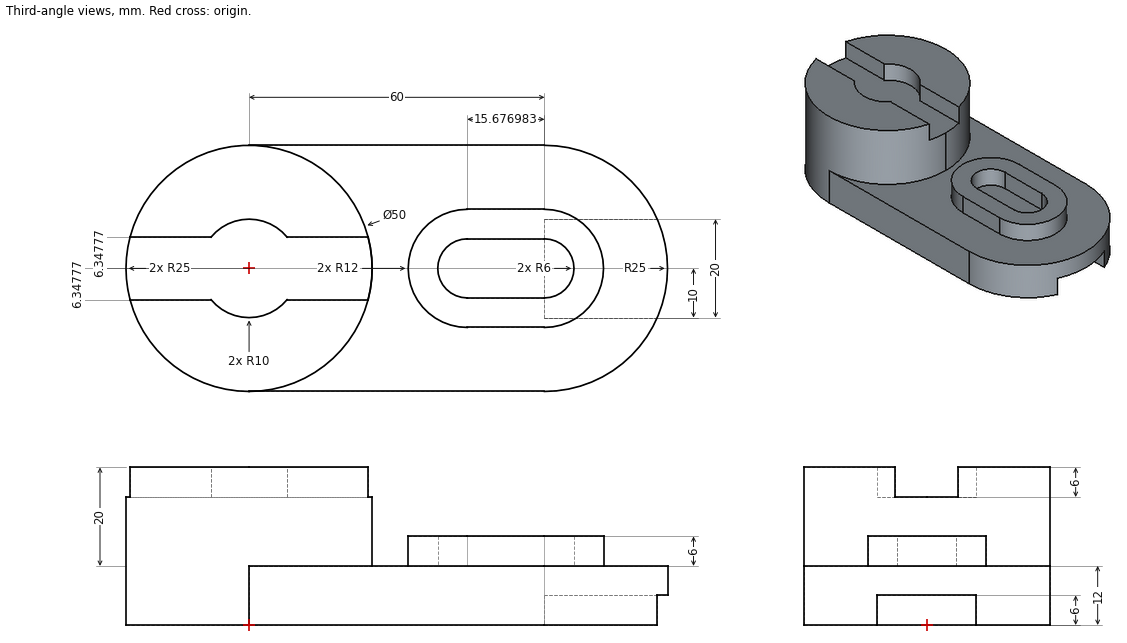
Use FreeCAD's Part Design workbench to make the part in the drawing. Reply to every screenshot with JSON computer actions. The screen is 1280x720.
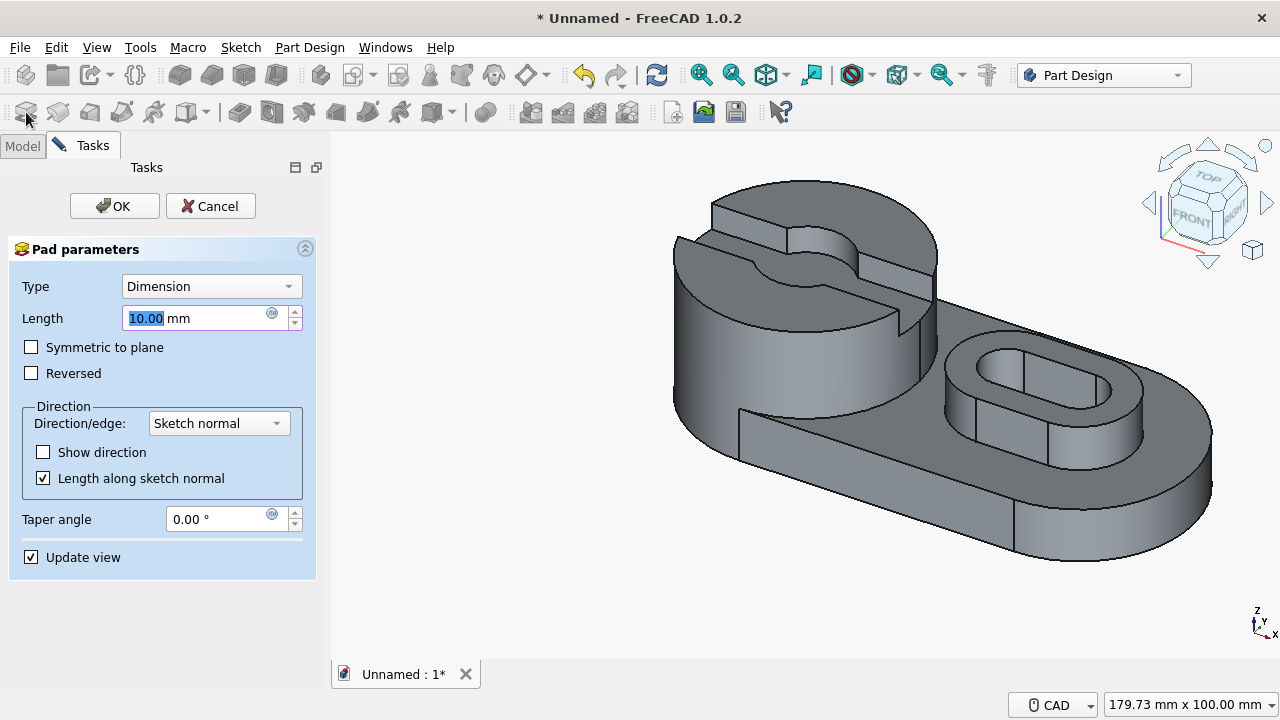
{"action": "type", "text": "6"}
{"action": "key", "text": "Tab"}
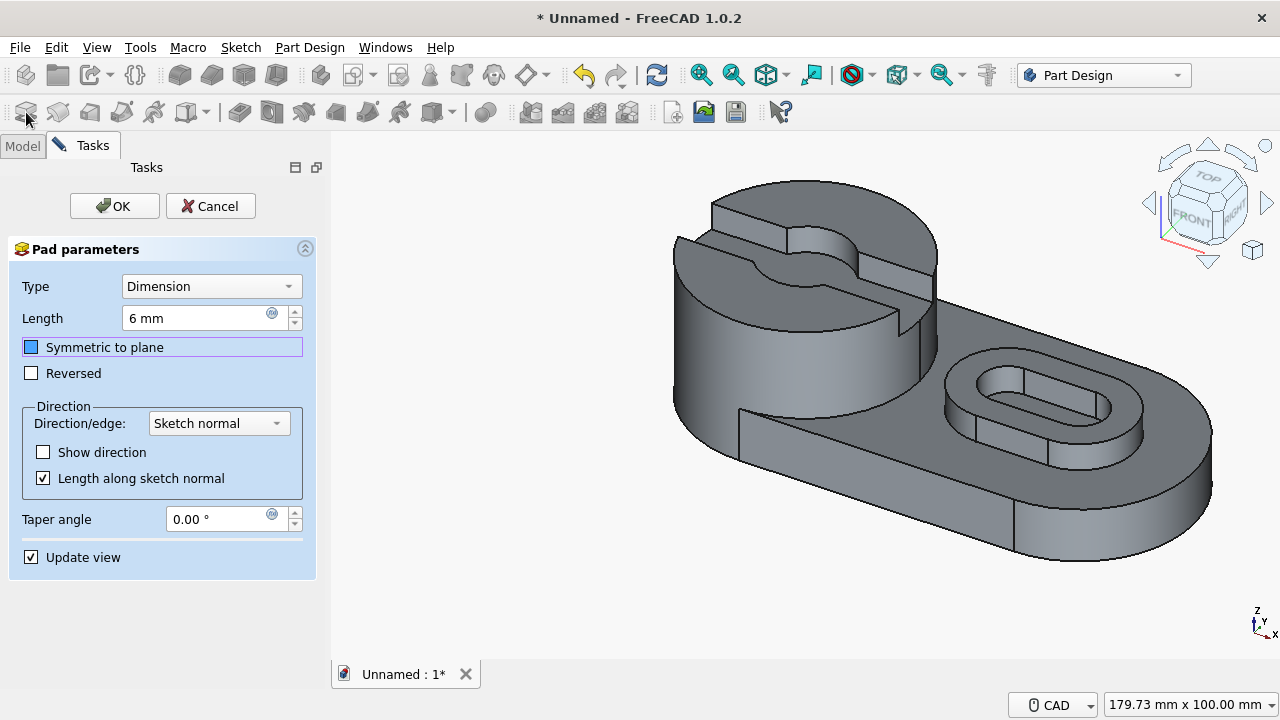
{"action": "left_click", "coordinate": [115, 206]}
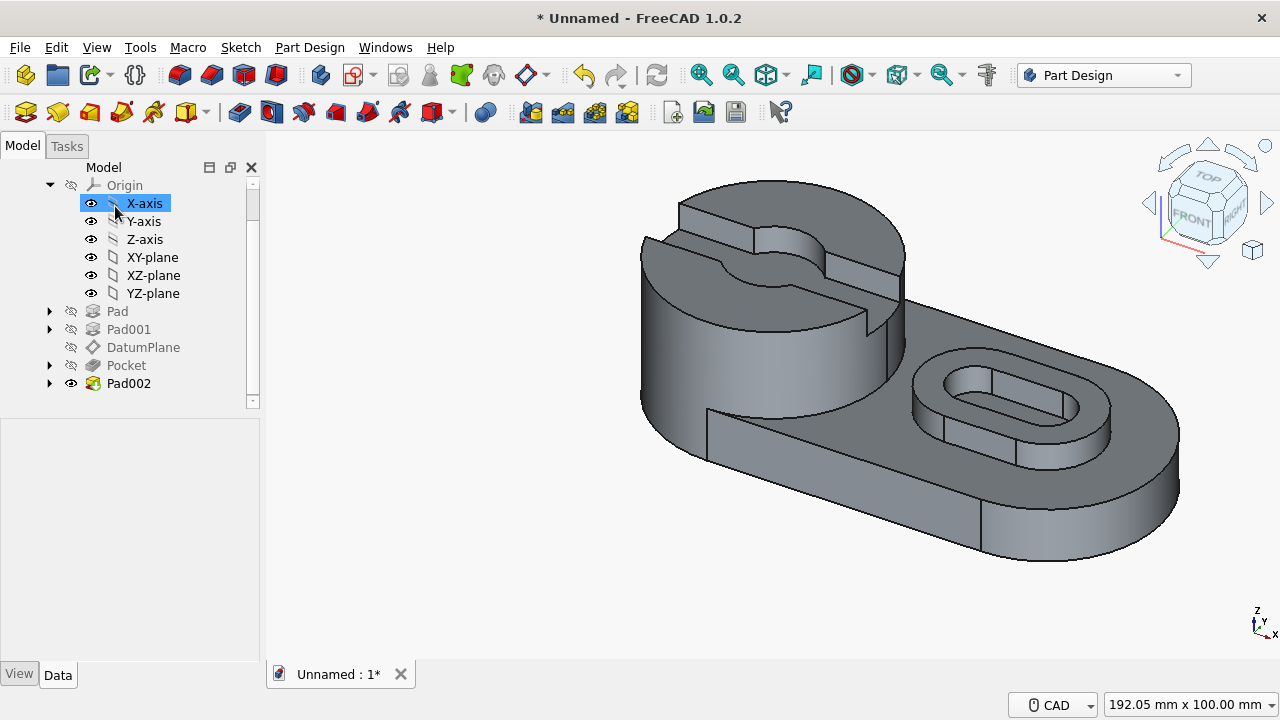
{"action": "key", "text": "5"}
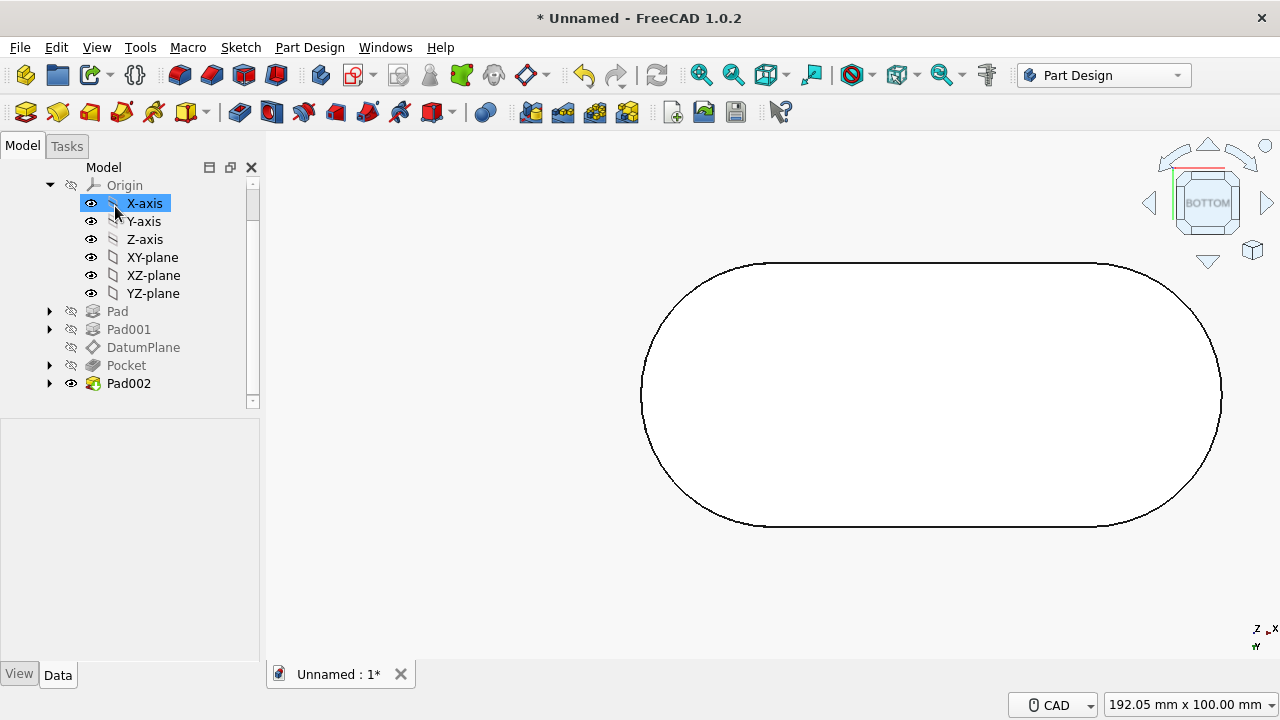
{"action": "left_click", "coordinate": [1014, 394]}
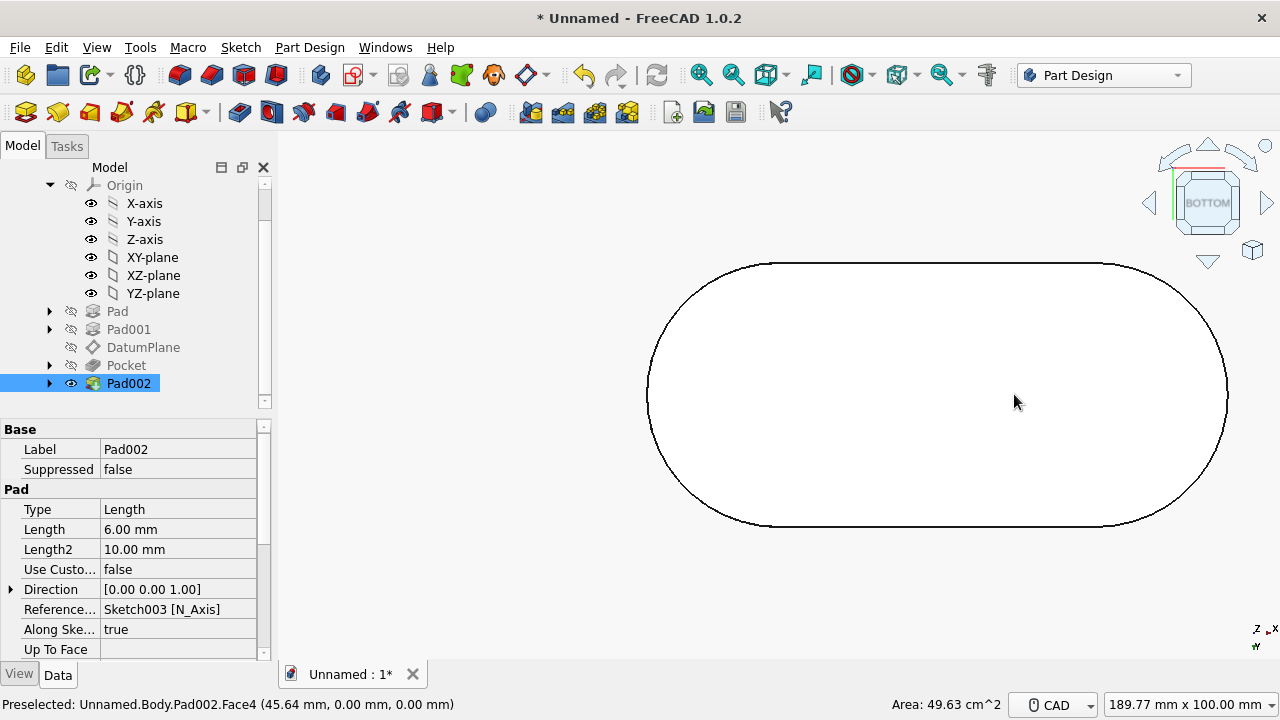
{"action": "left_click", "coordinate": [354, 76]}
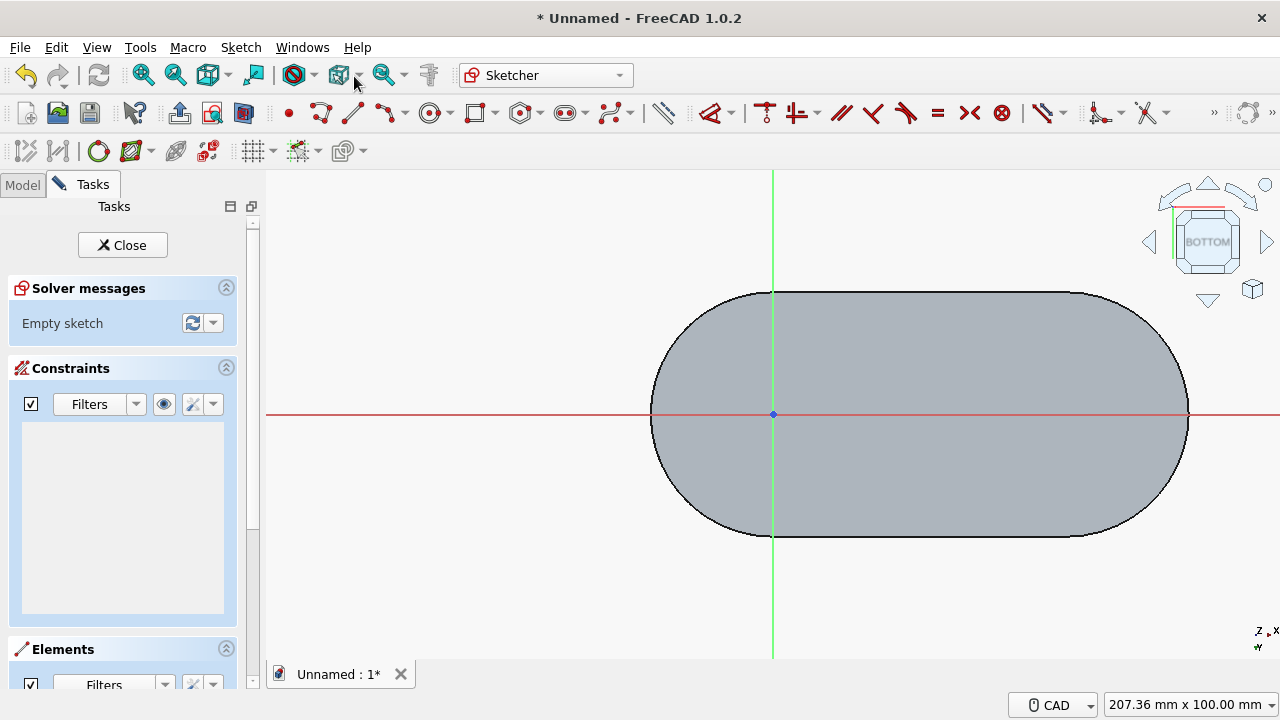
{"action": "scroll", "coordinate": [704, 414], "scroll_direction": "down", "scroll_amount": 5}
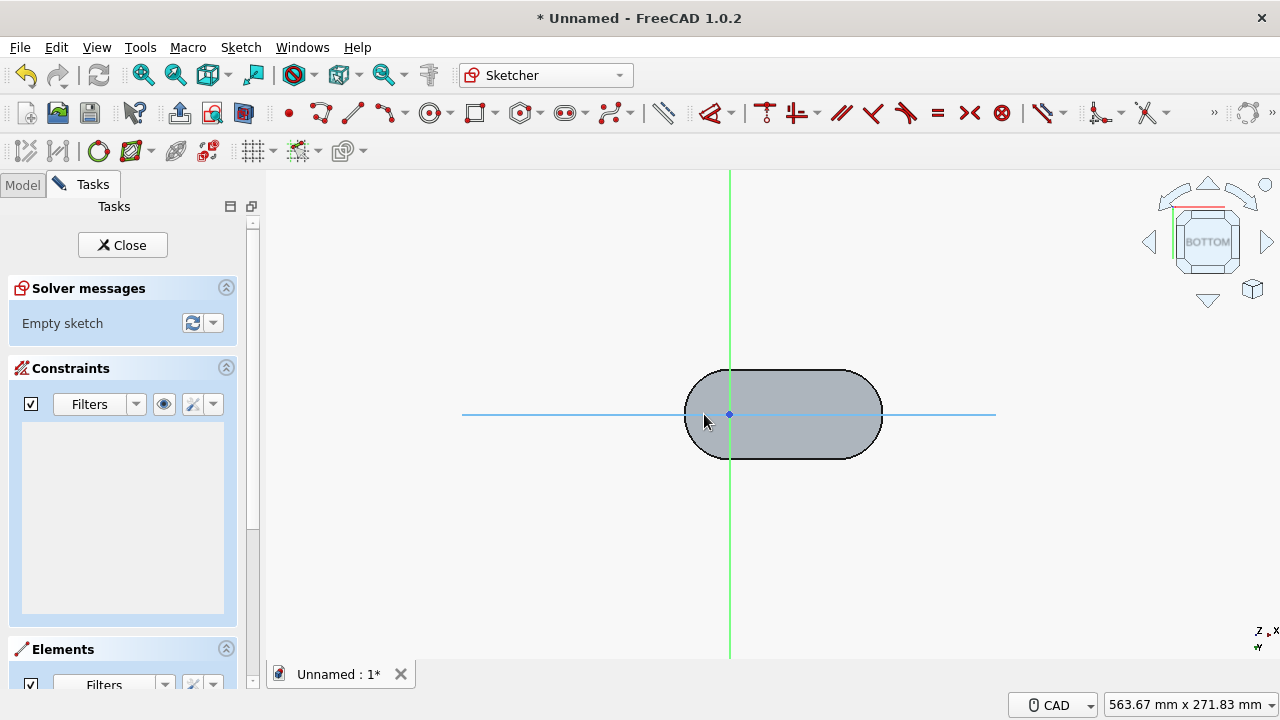
{"action": "scroll", "coordinate": [879, 414], "scroll_direction": "up", "scroll_amount": 11}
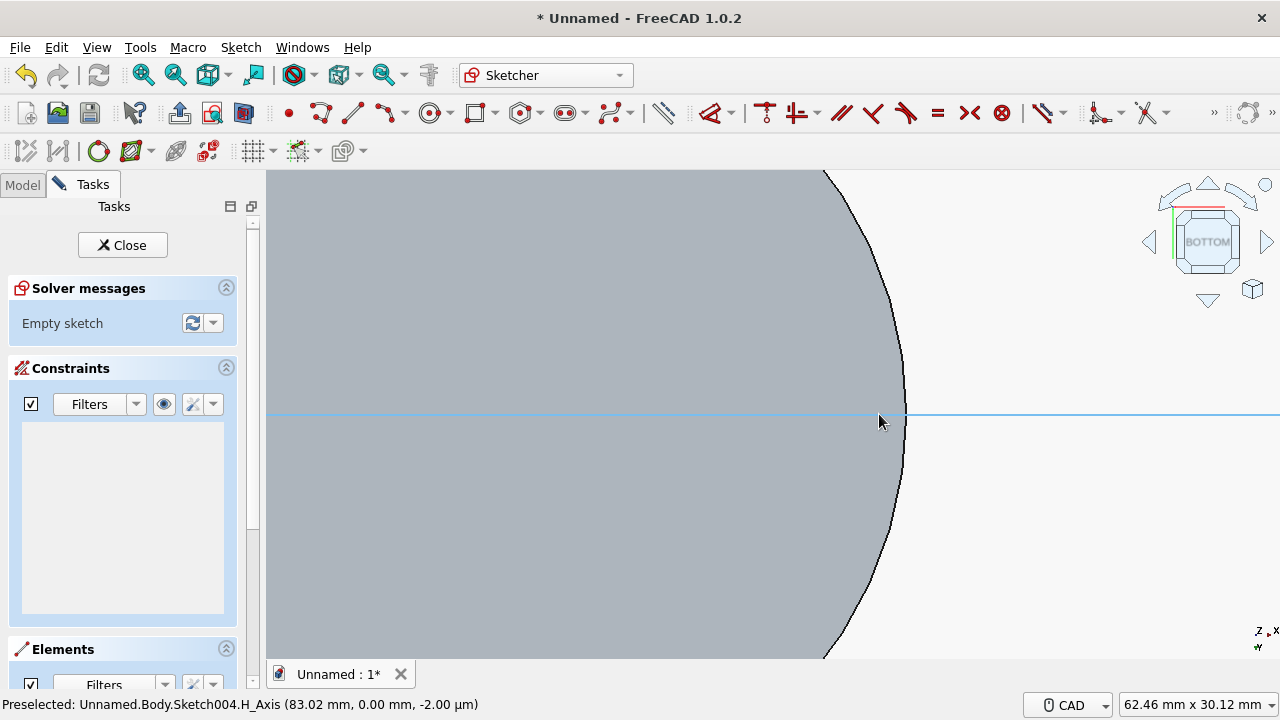
{"action": "left_click", "coordinate": [322, 114]}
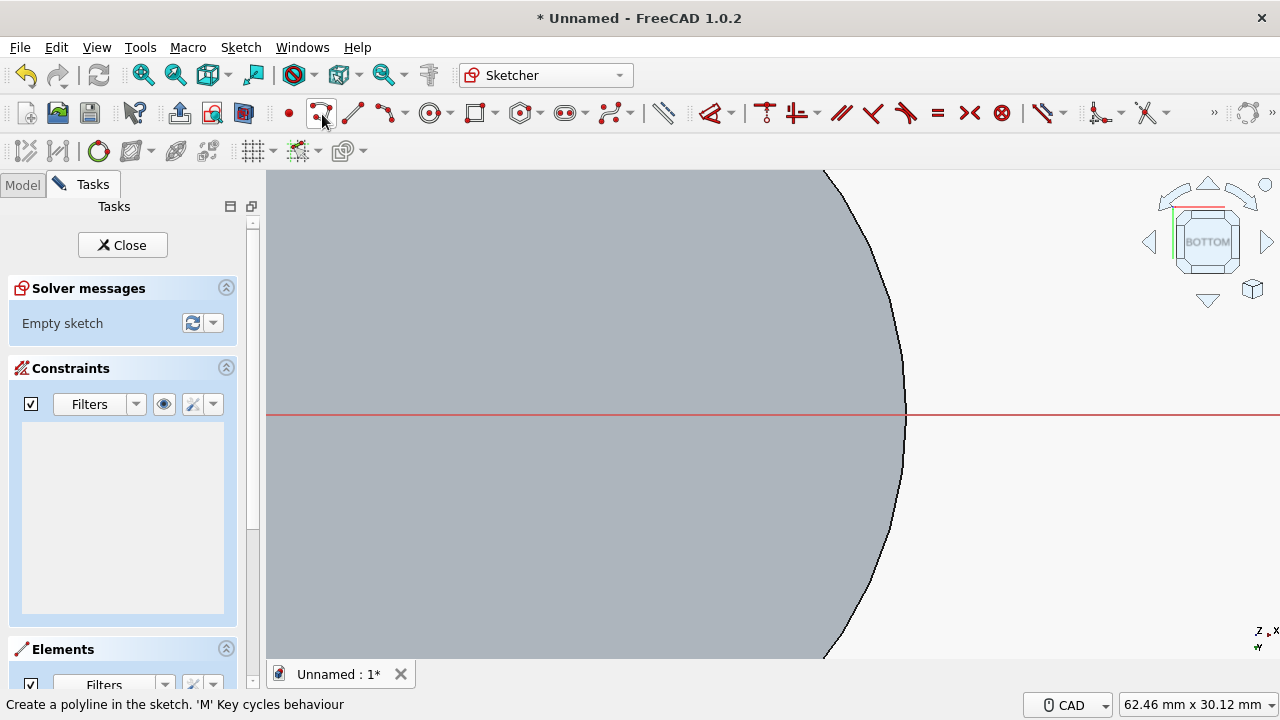
{"action": "left_click", "coordinate": [872, 252]}
{"action": "left_click", "coordinate": [500, 252]}
{"action": "left_click", "coordinate": [500, 577]}
{"action": "left_click", "coordinate": [872, 577]}
{"action": "right_click", "coordinate": [872, 577]}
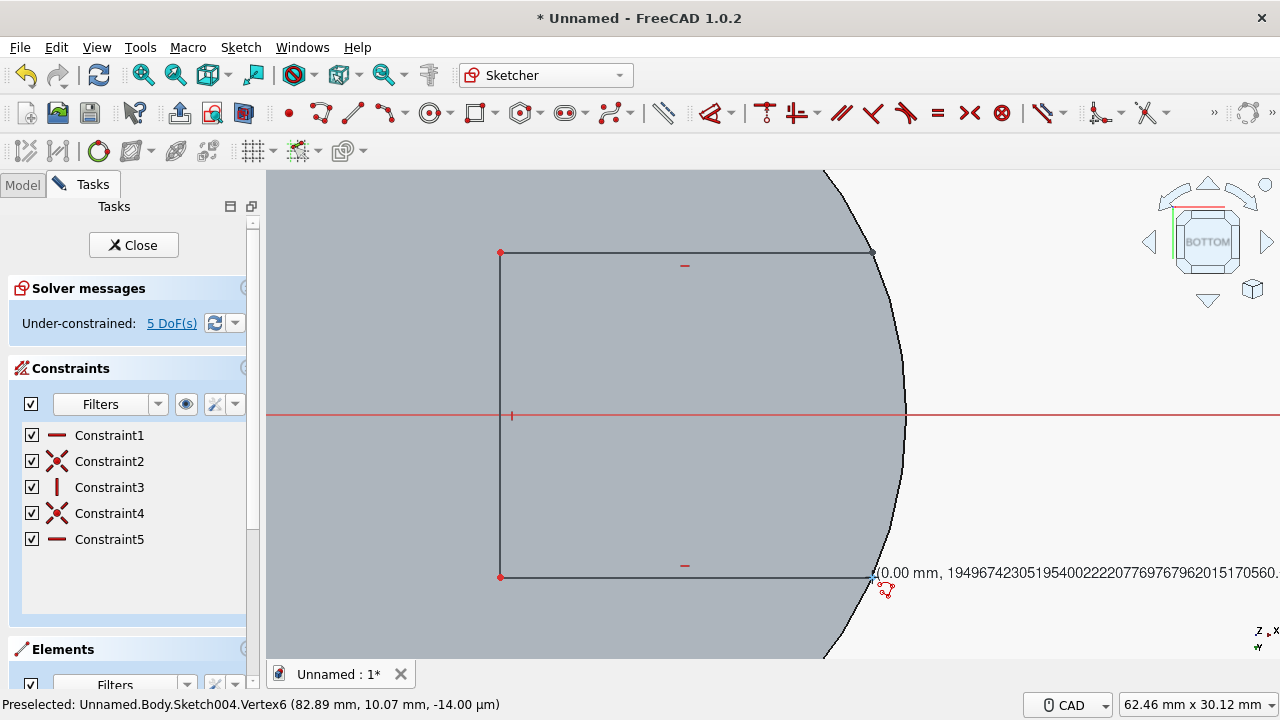
{"action": "key", "text": "g 3 a"}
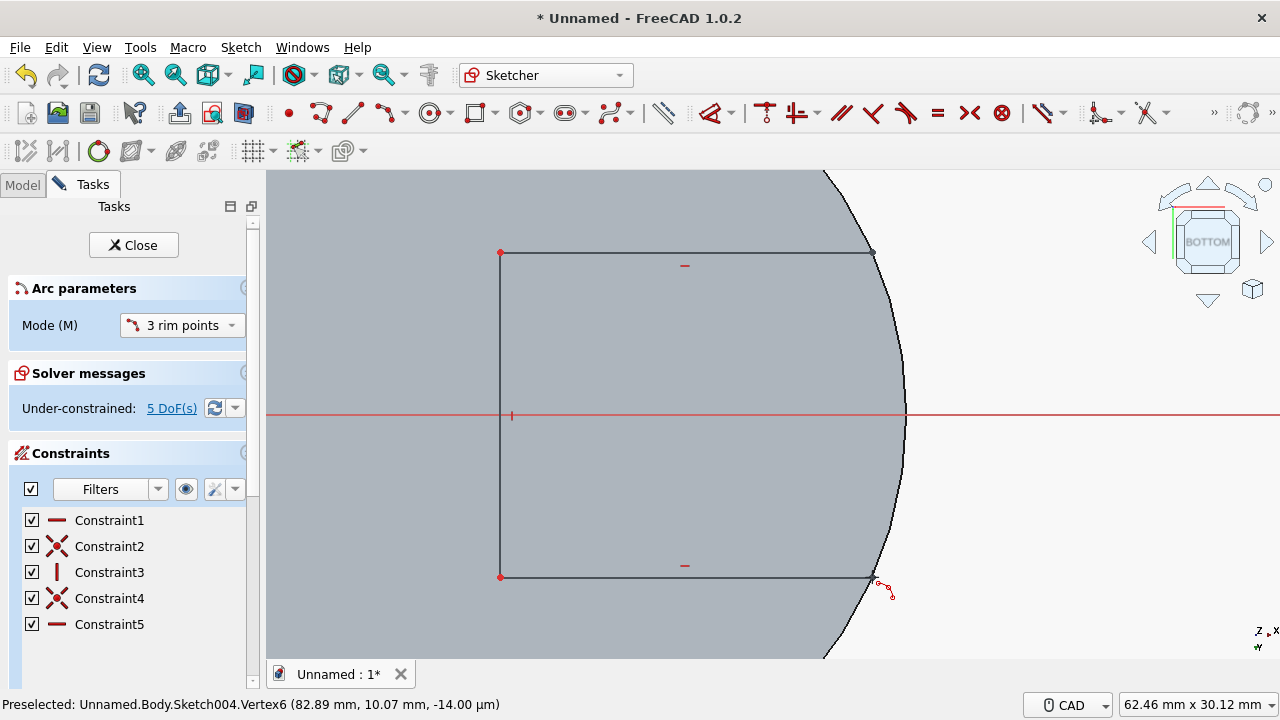
{"action": "left_click", "coordinate": [872, 578]}
{"action": "left_click", "coordinate": [872, 253]}
{"action": "left_click", "coordinate": [905, 448]}
{"action": "key", "text": "Escape"}